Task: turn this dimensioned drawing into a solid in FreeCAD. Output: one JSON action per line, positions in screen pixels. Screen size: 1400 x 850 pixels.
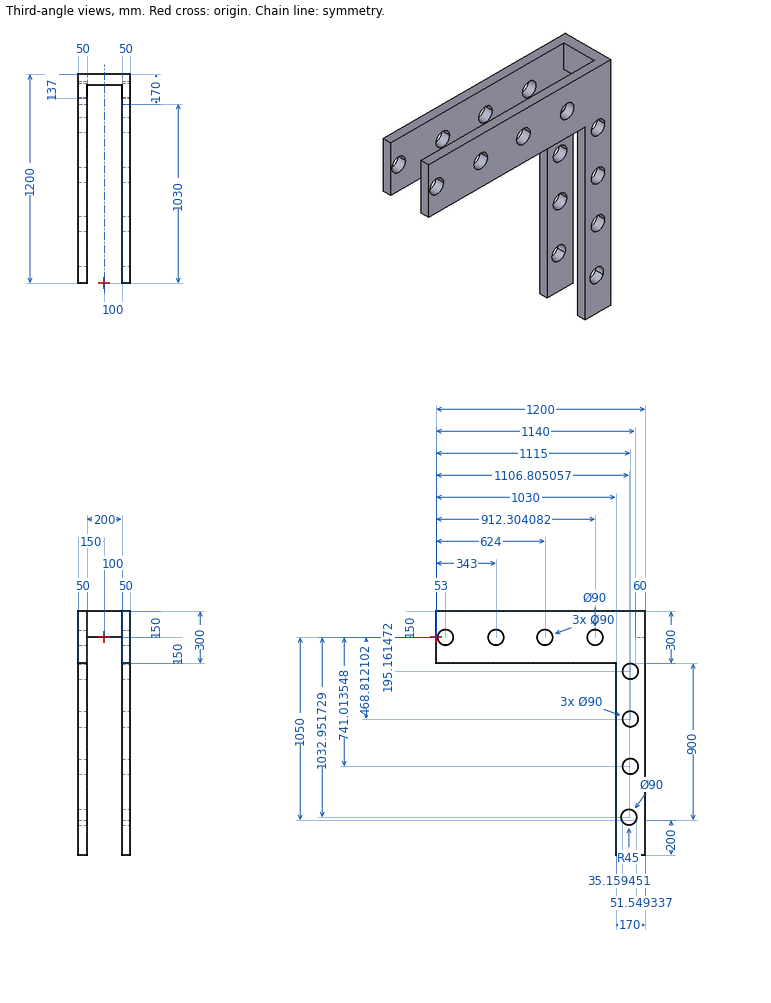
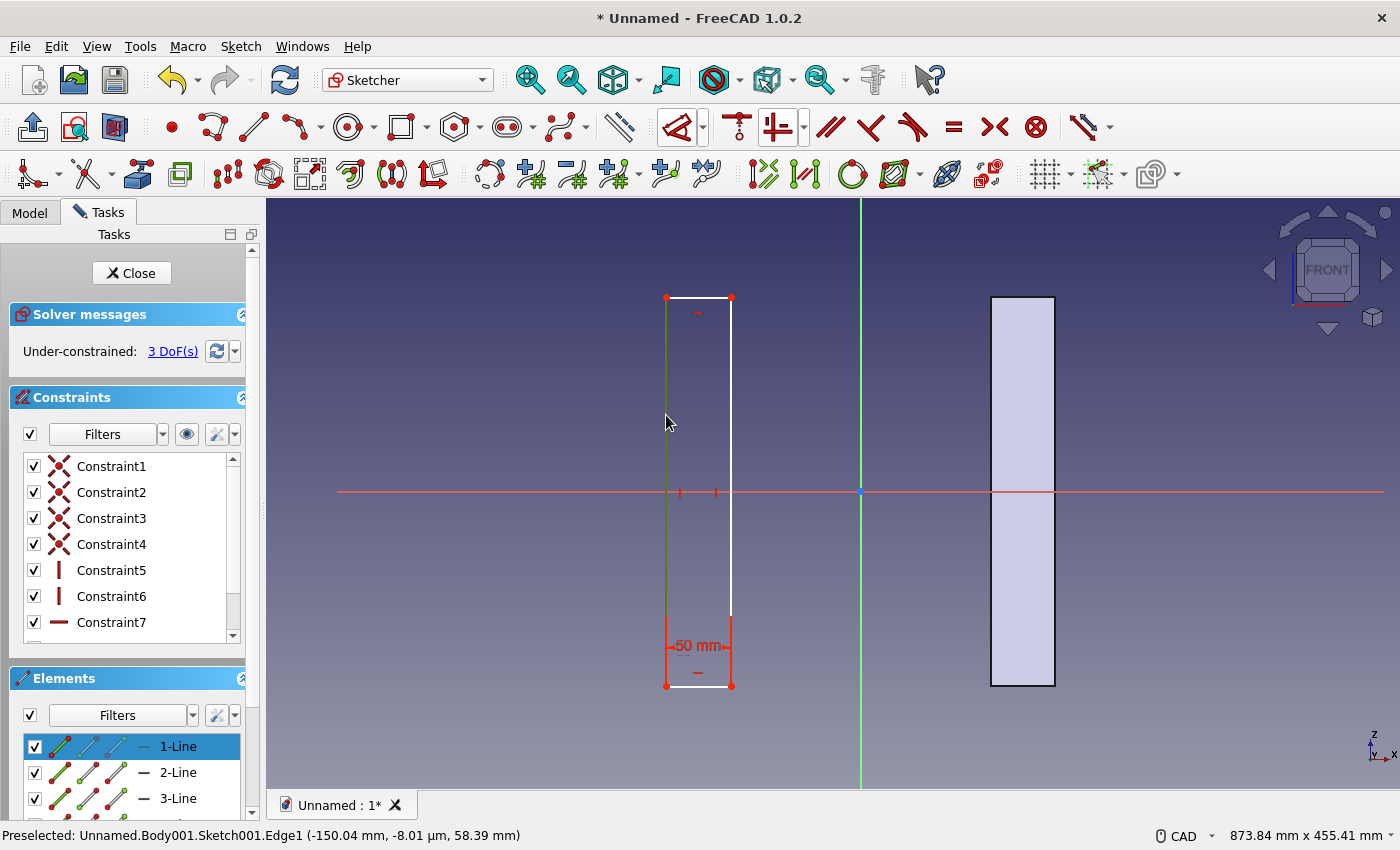
{"action": "left_click", "coordinate": [702, 128]}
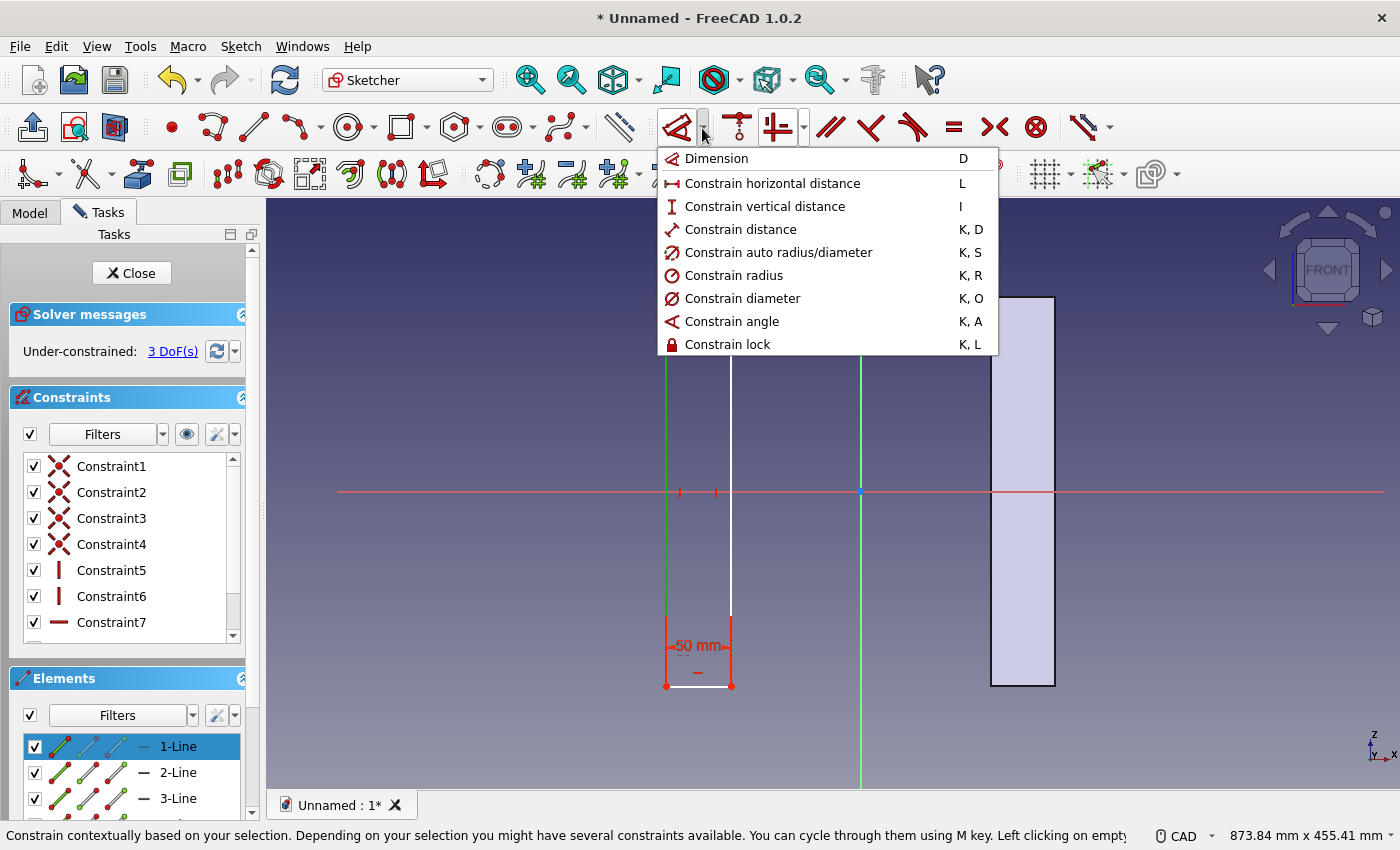
{"action": "left_click", "coordinate": [828, 206]}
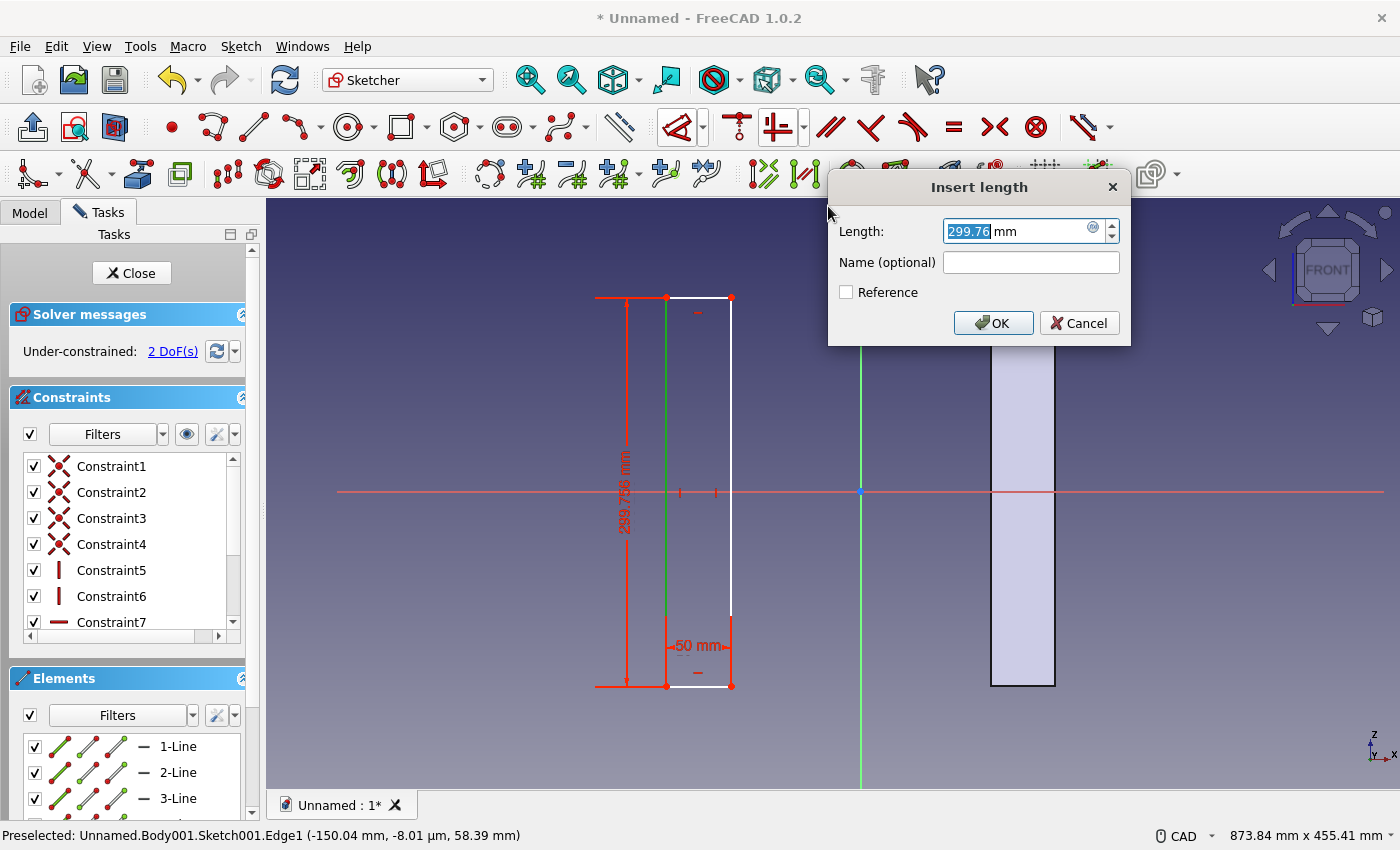
{"action": "type", "text": "300"}
{"action": "key", "text": "Return"}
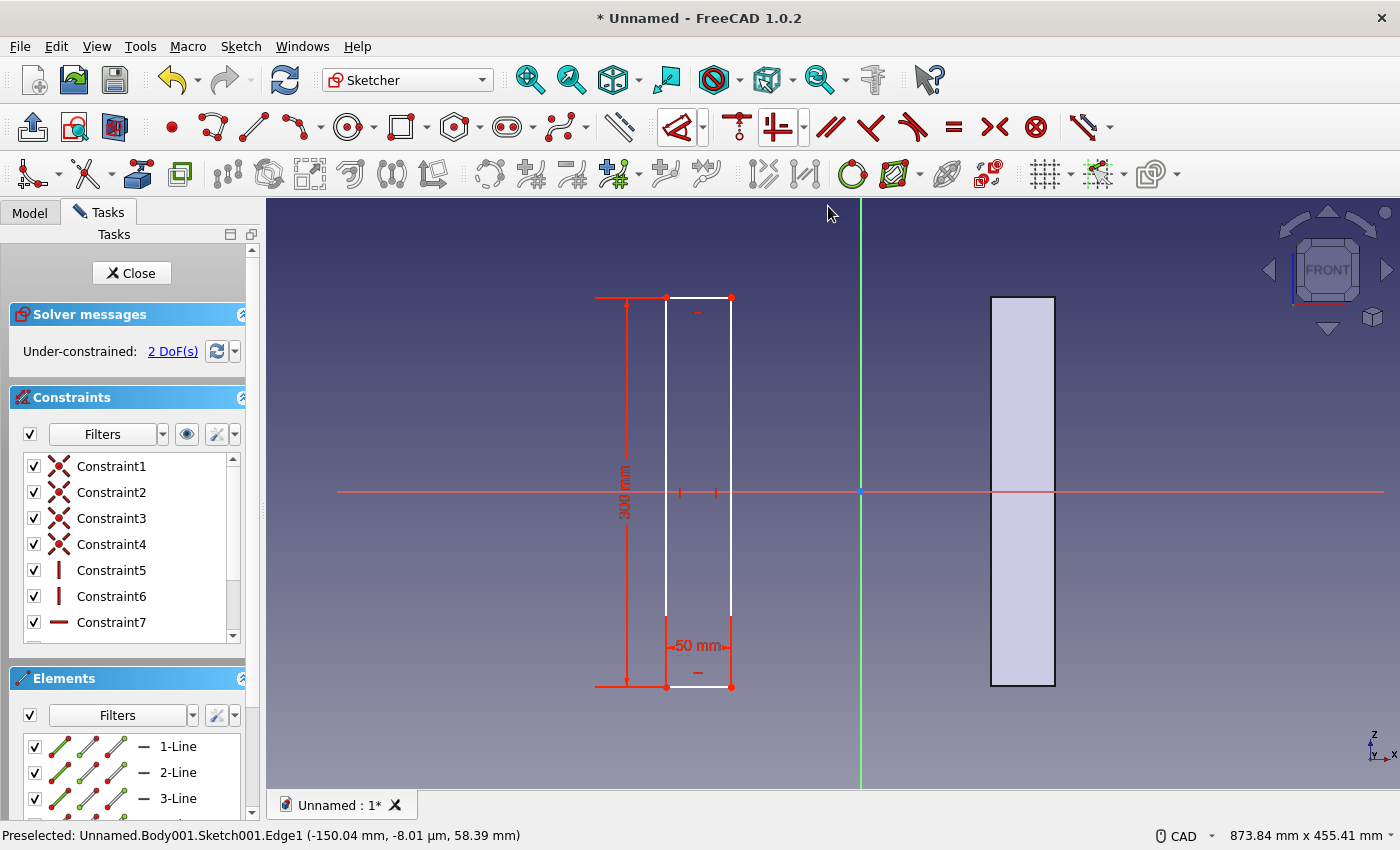
{"action": "left_click", "coordinate": [666, 298]}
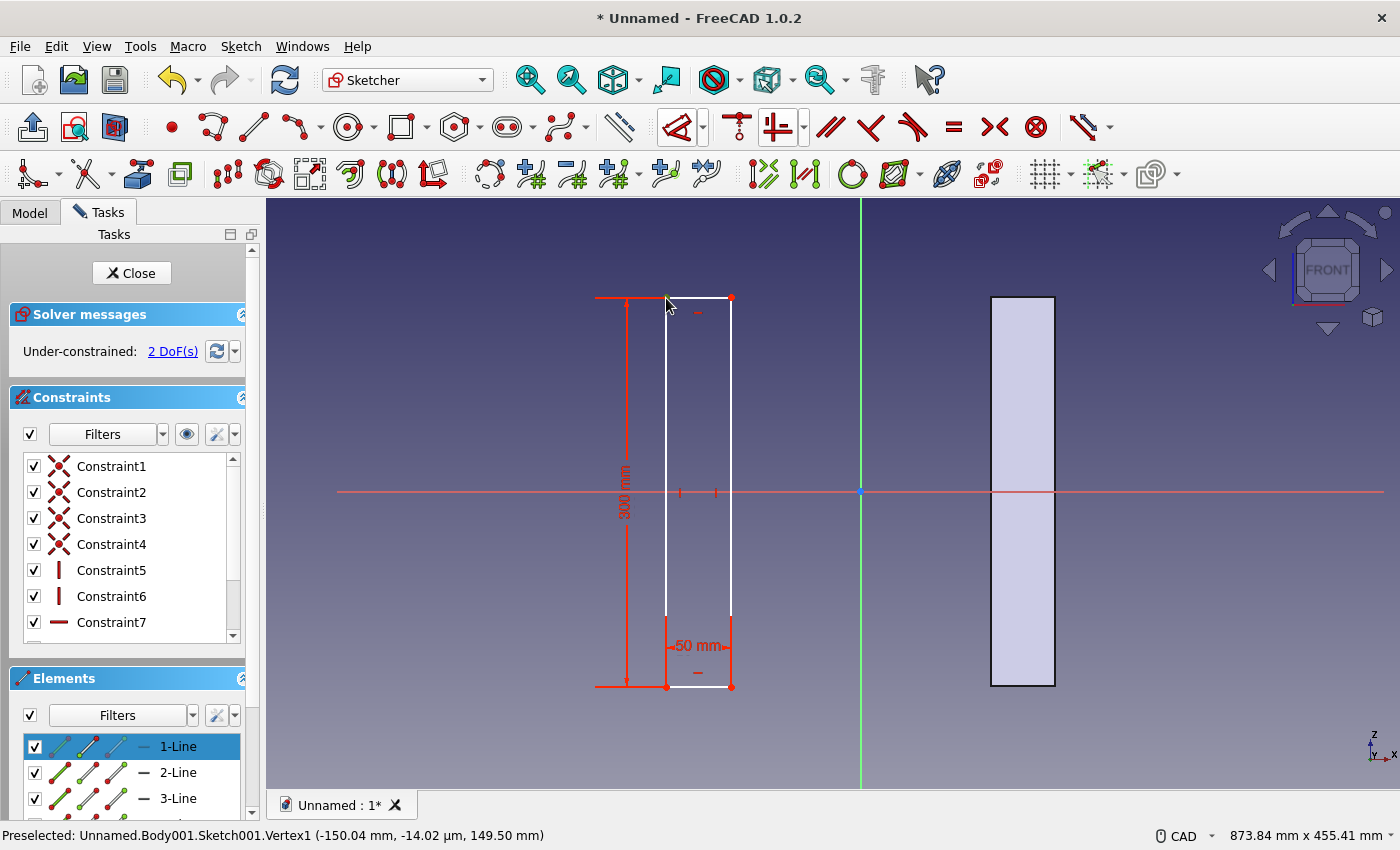
{"action": "left_click", "coordinate": [702, 128]}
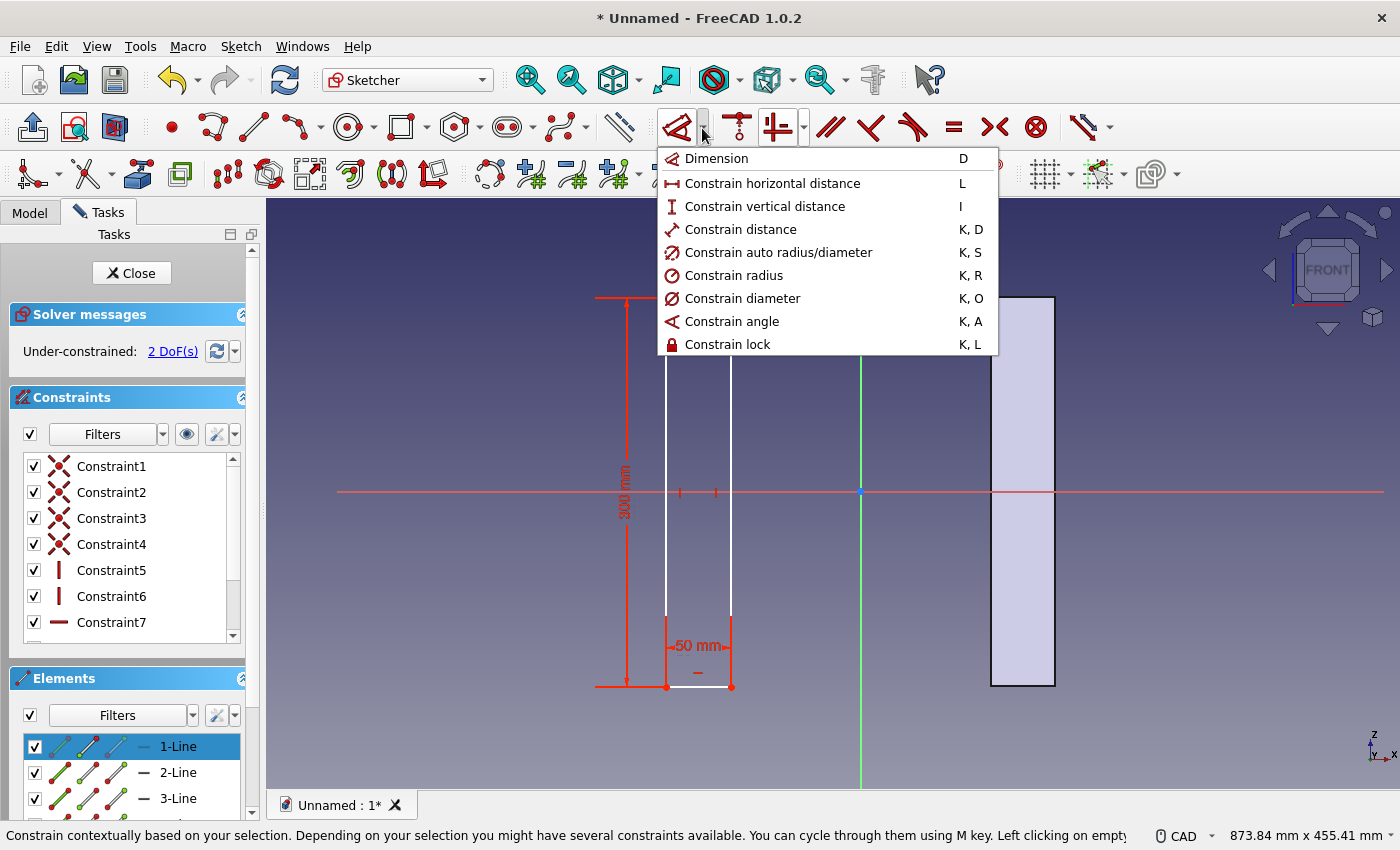
{"action": "left_click", "coordinate": [828, 184]}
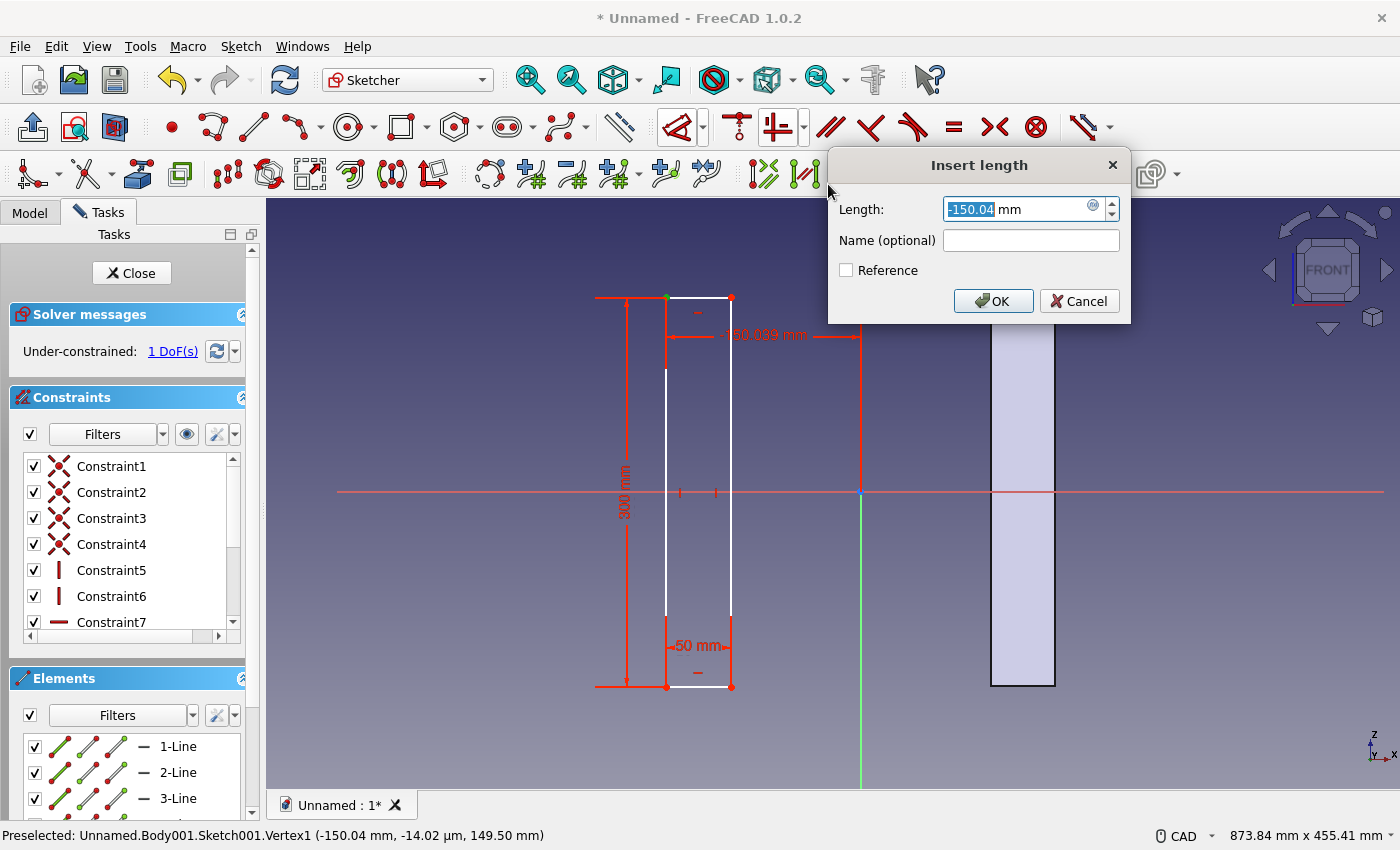
{"action": "type", "text": "-150"}
{"action": "key", "text": "Return"}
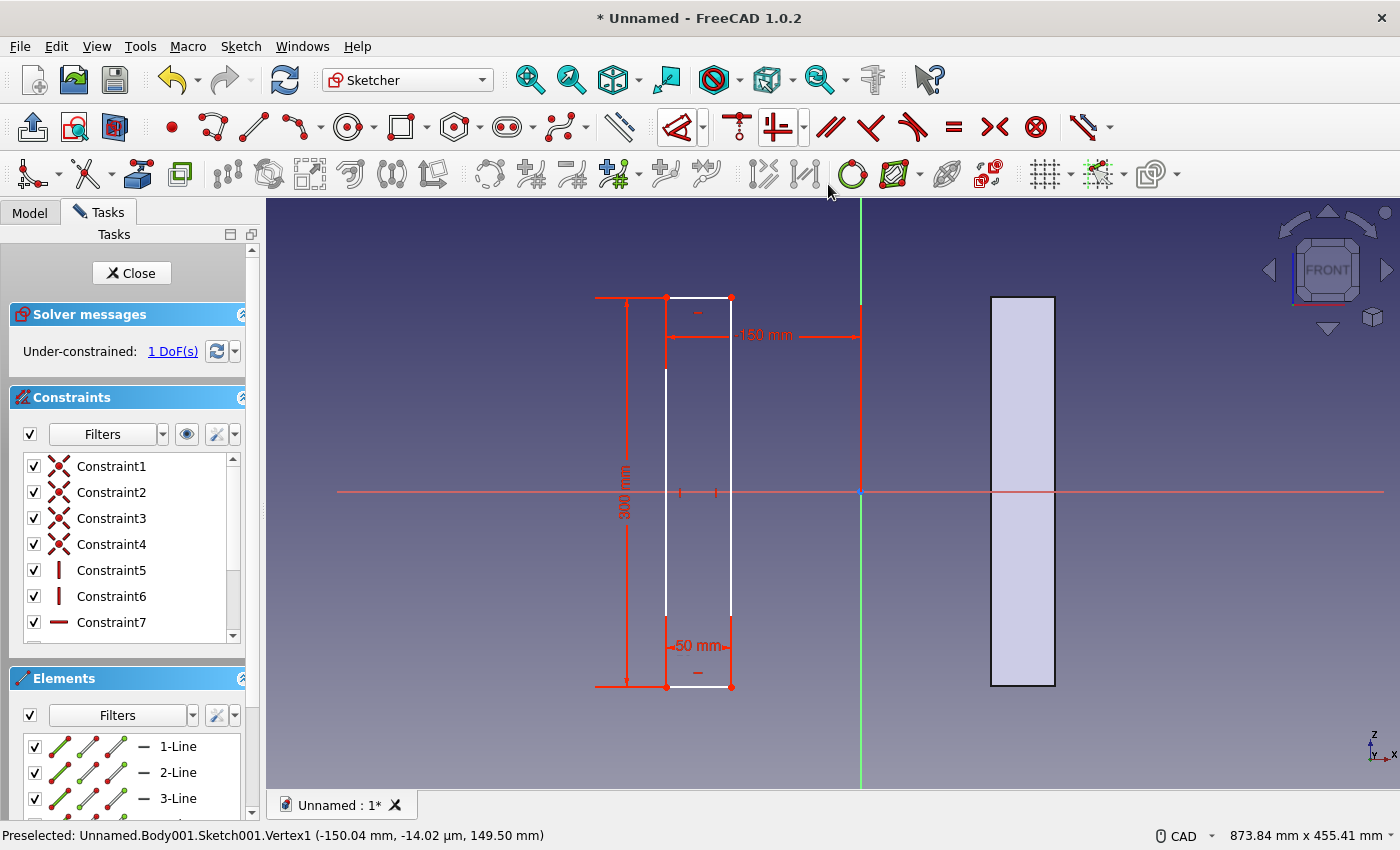
{"action": "left_click", "coordinate": [666, 298]}